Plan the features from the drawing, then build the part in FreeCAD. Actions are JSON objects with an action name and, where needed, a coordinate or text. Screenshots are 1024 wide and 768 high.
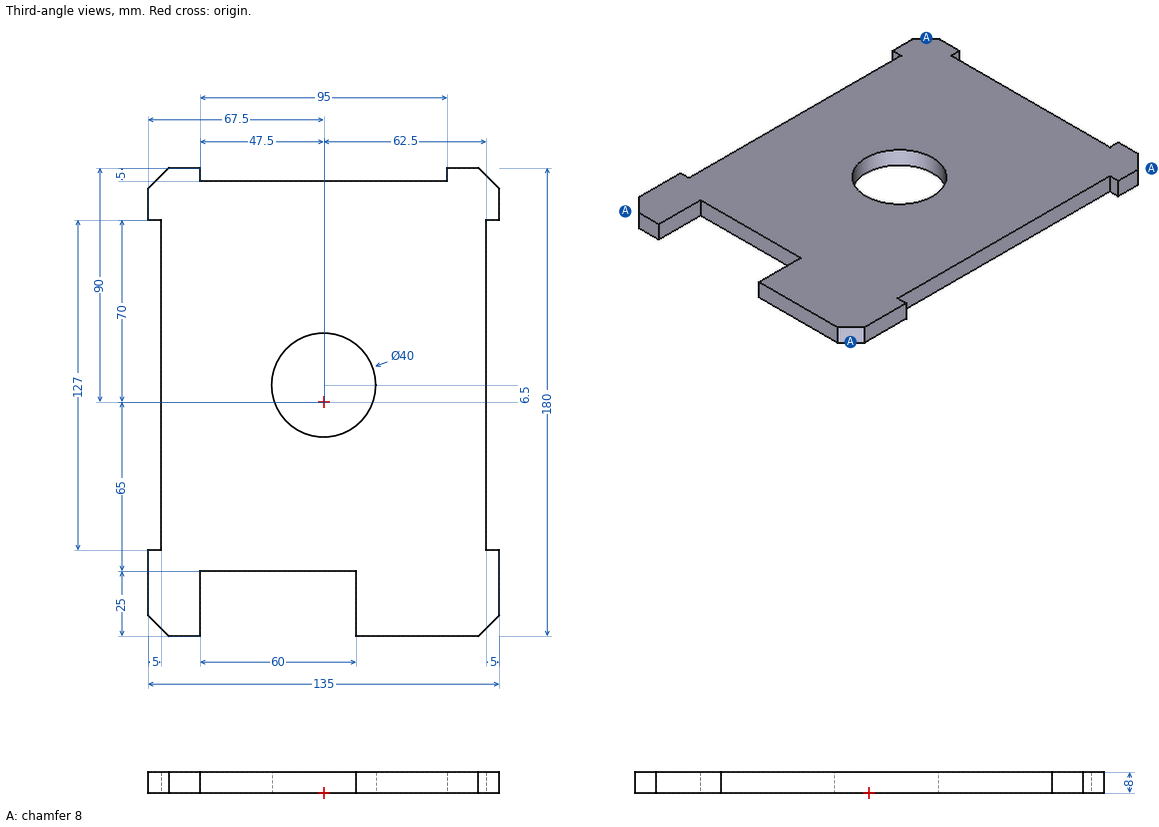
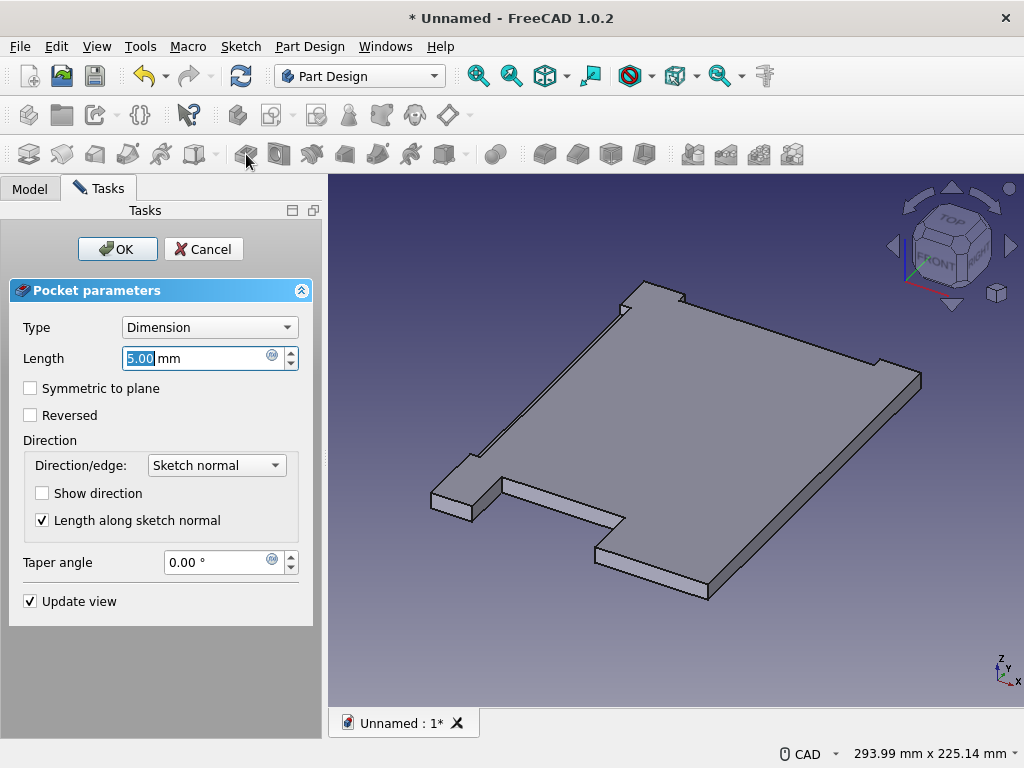
{"action": "left_click", "coordinate": [210, 328]}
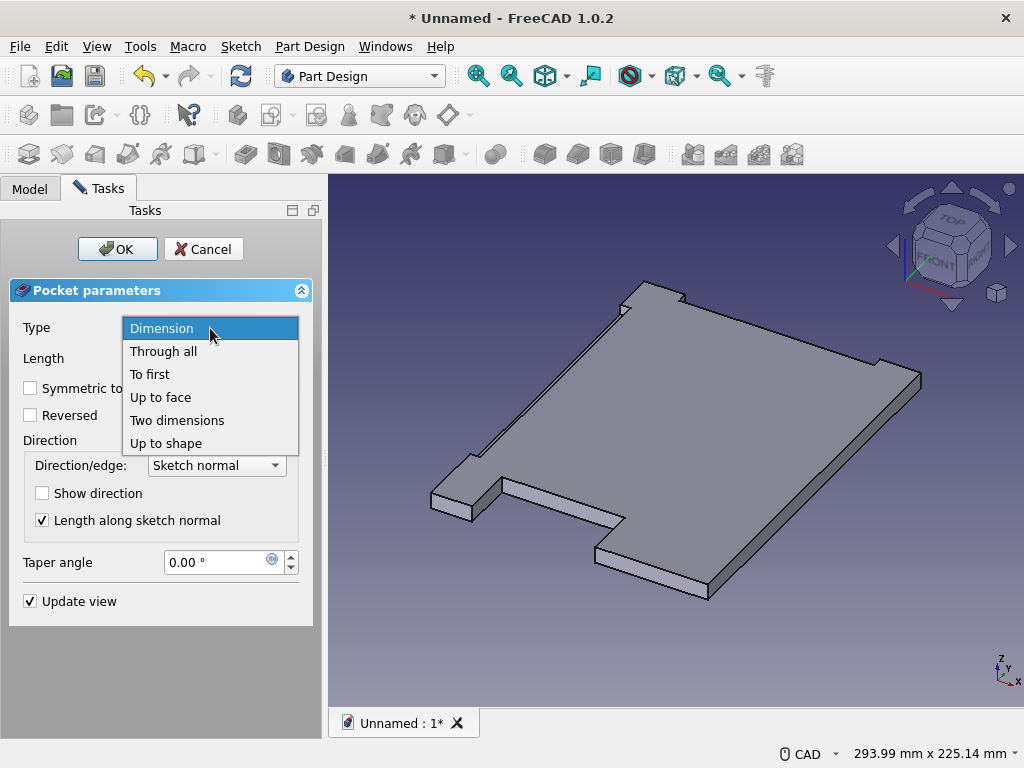
{"action": "left_click", "coordinate": [208, 374]}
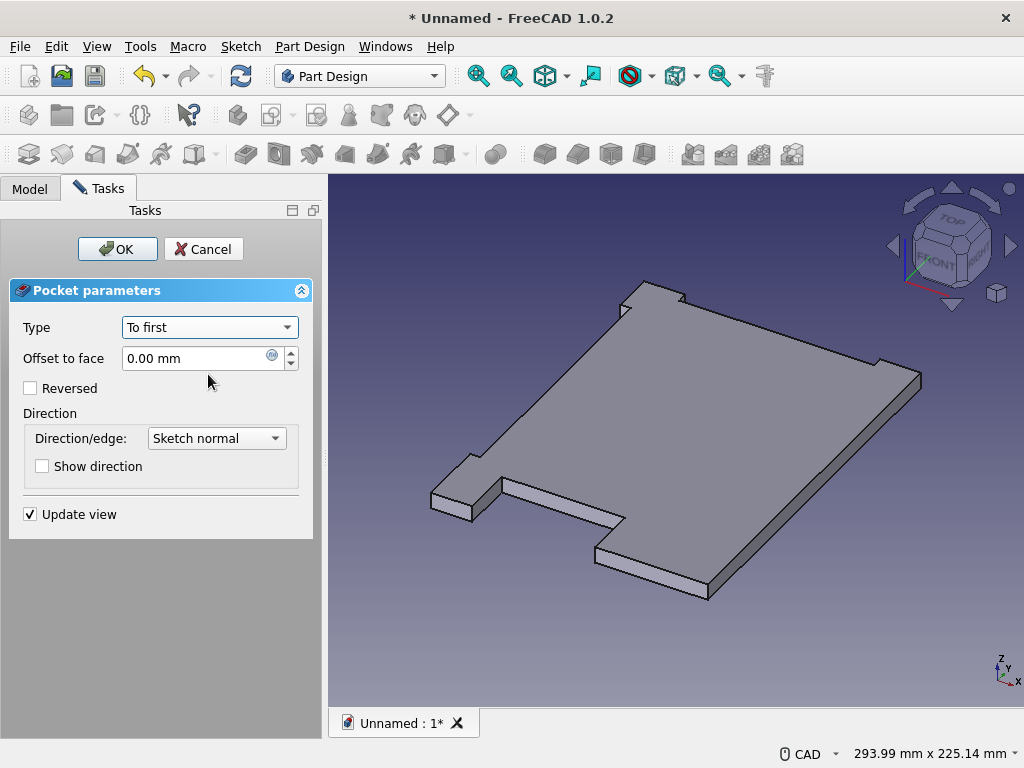
{"action": "left_click", "coordinate": [118, 249]}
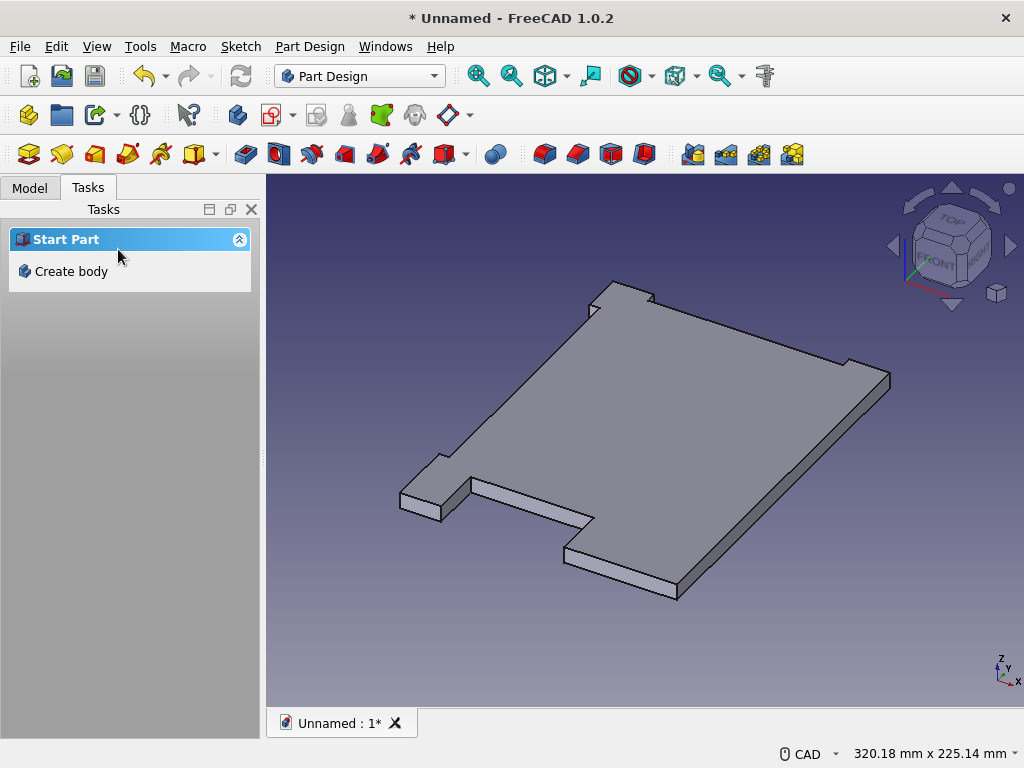
{"action": "left_click", "coordinate": [645, 432]}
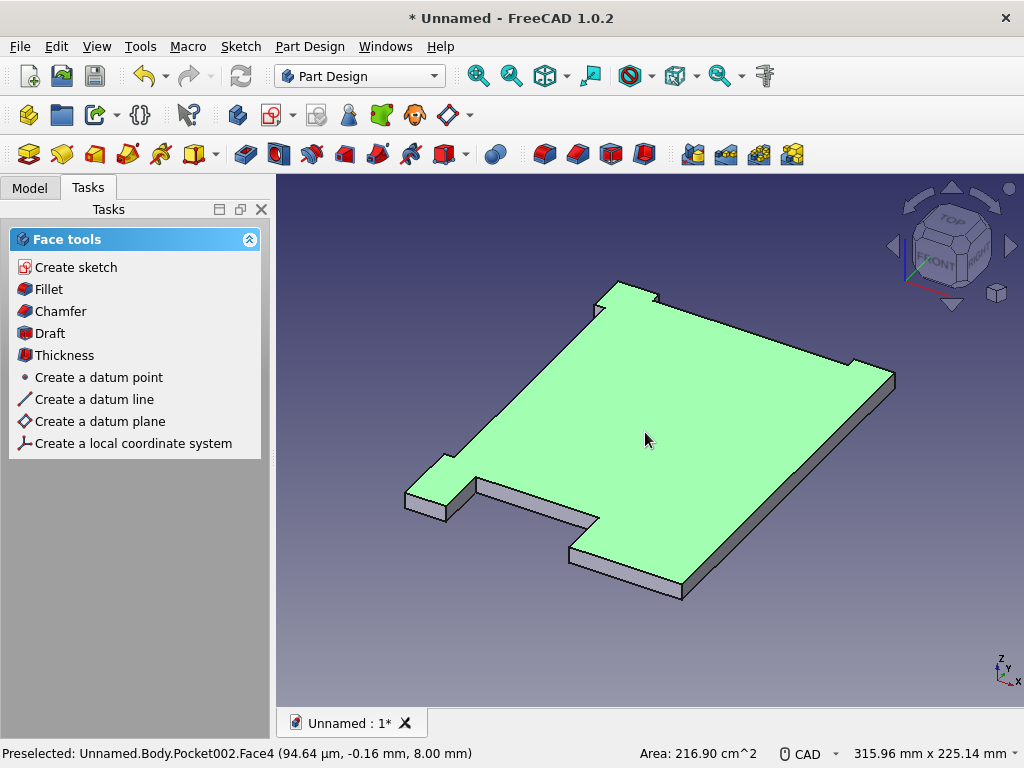
{"action": "left_click", "coordinate": [270, 116]}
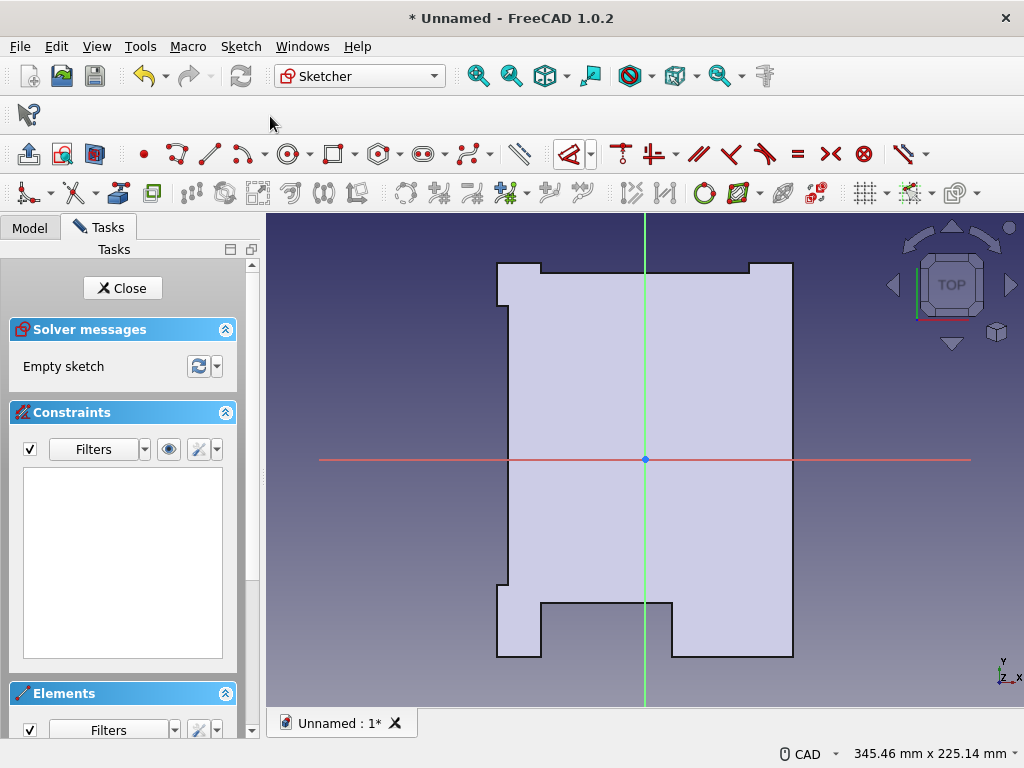
{"action": "key", "text": "g r"}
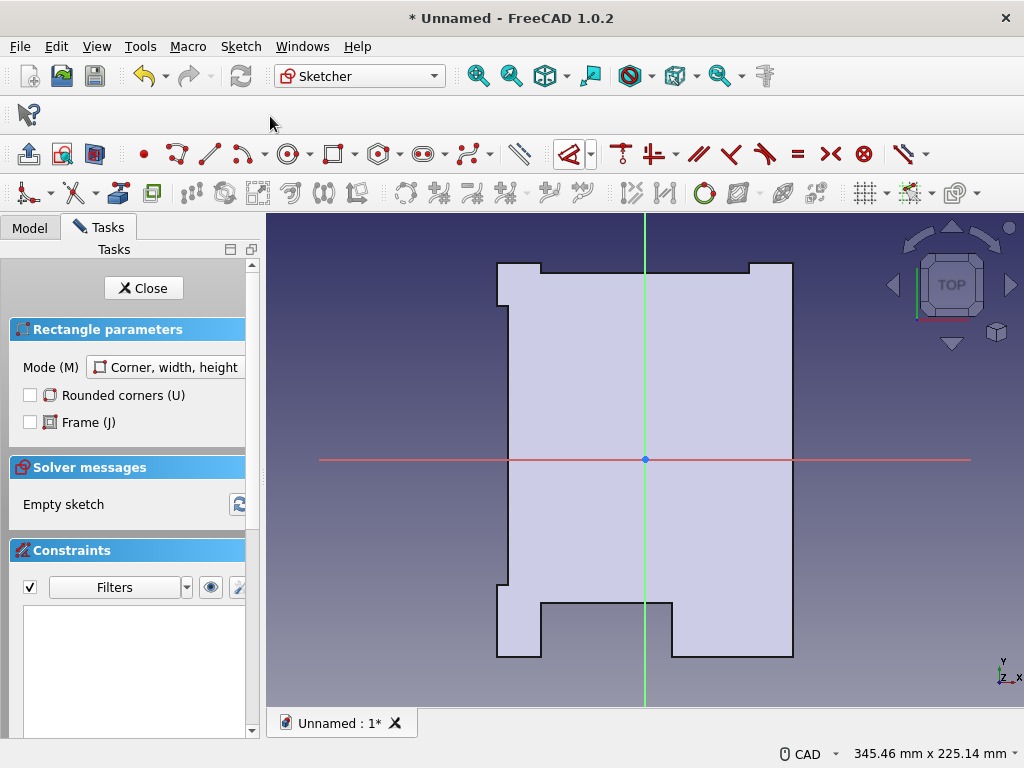
{"action": "scroll", "coordinate": [782, 306], "scroll_direction": "up", "scroll_amount": 2}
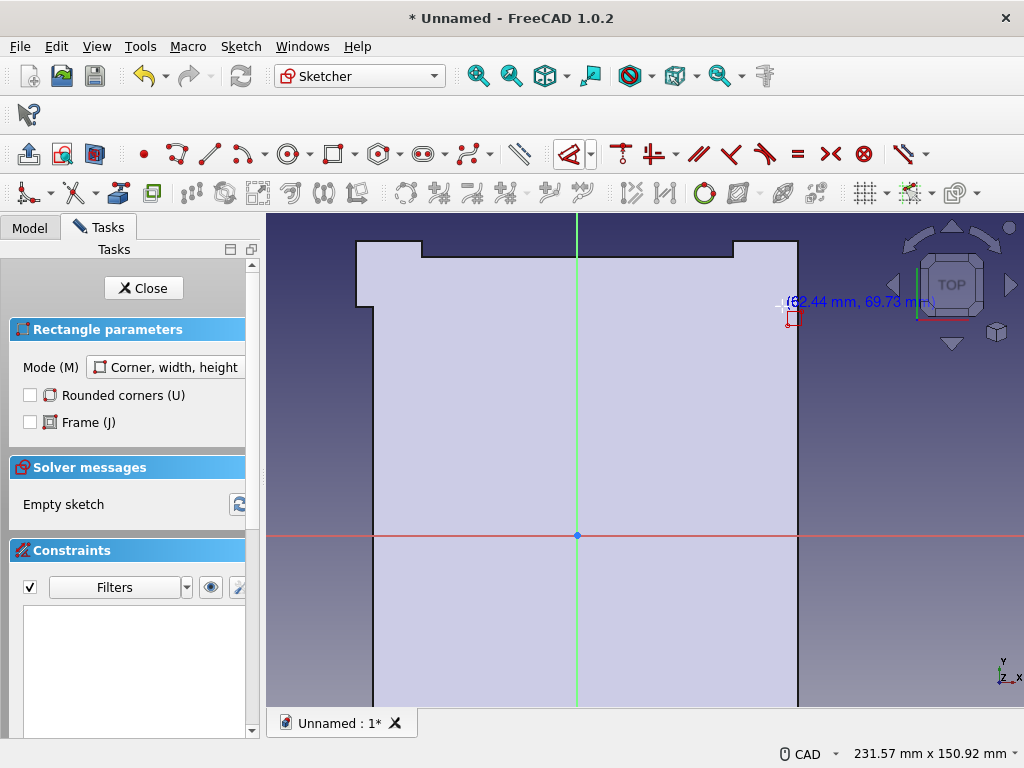
{"action": "left_click", "coordinate": [782, 307]}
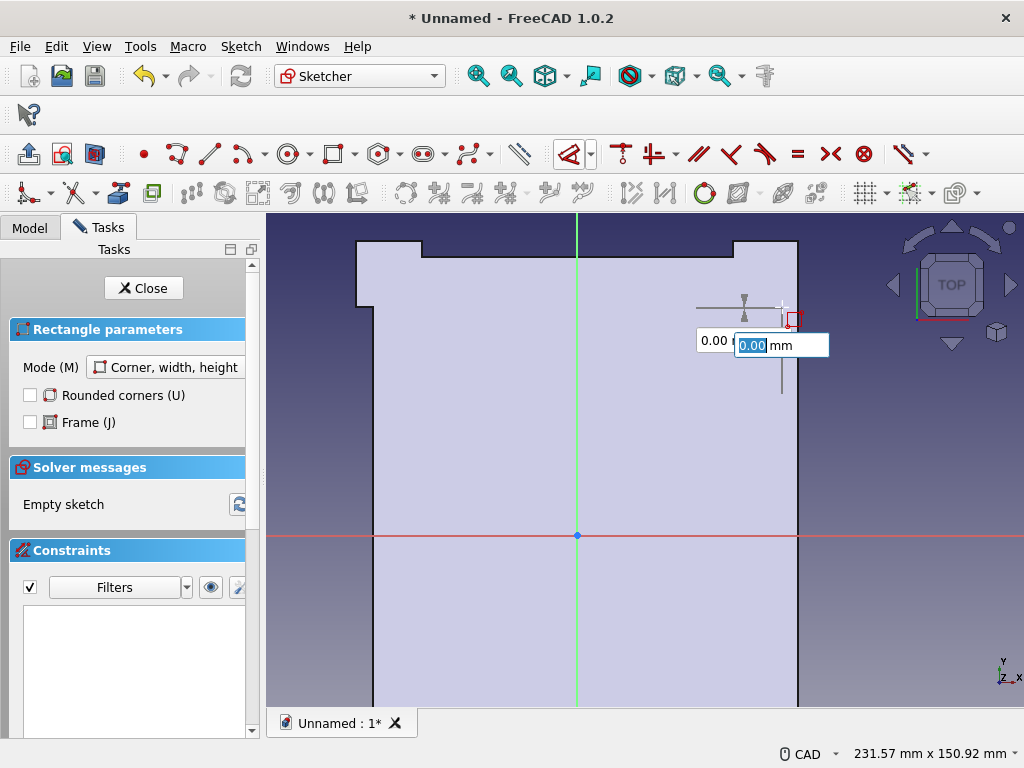
{"action": "scroll", "coordinate": [294, 241], "scroll_direction": "down", "scroll_amount": 1}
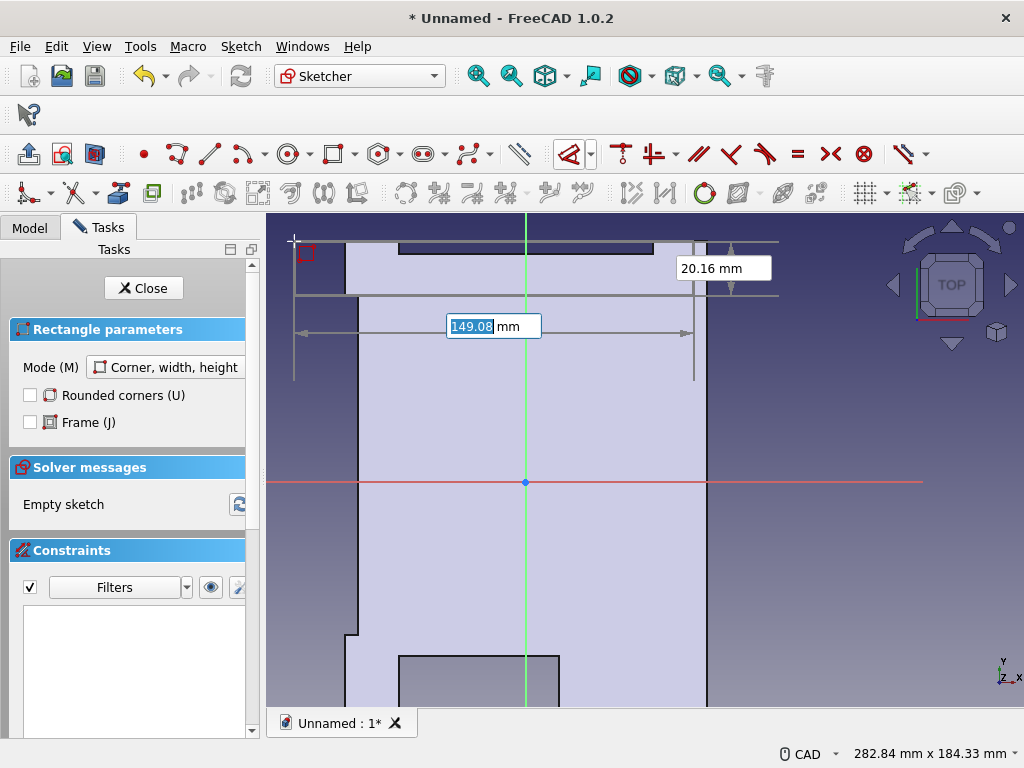
{"action": "left_click", "coordinate": [707, 635]}
{"action": "key", "text": "Escape"}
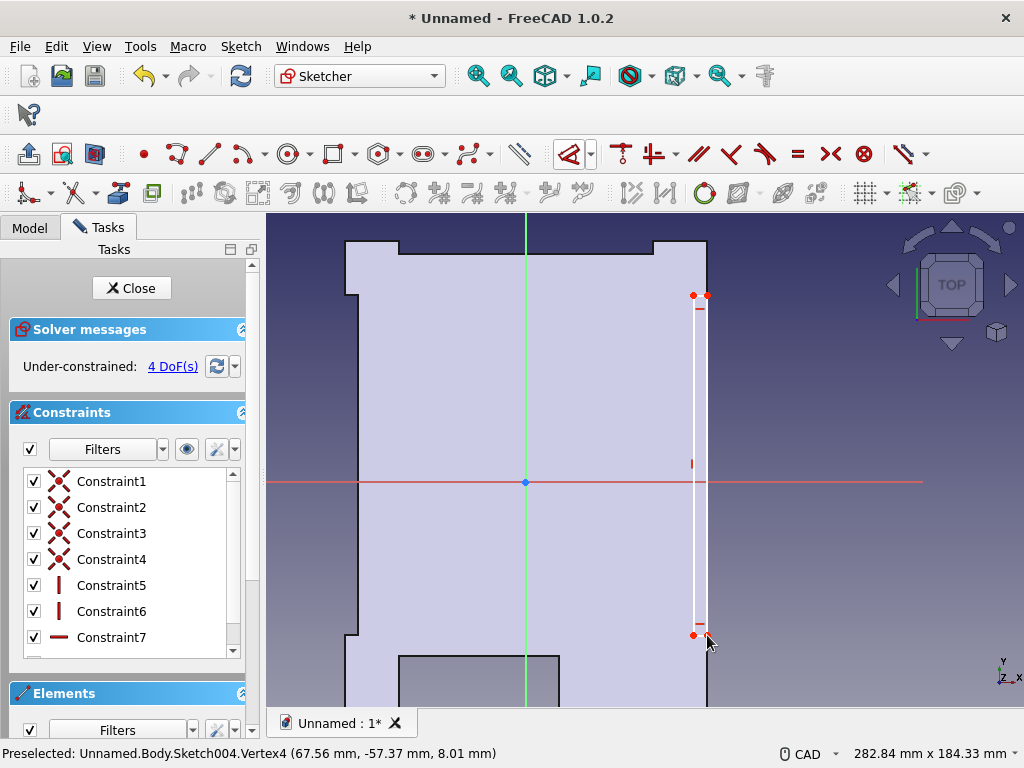
{"action": "scroll", "coordinate": [700, 636], "scroll_direction": "up", "scroll_amount": 6}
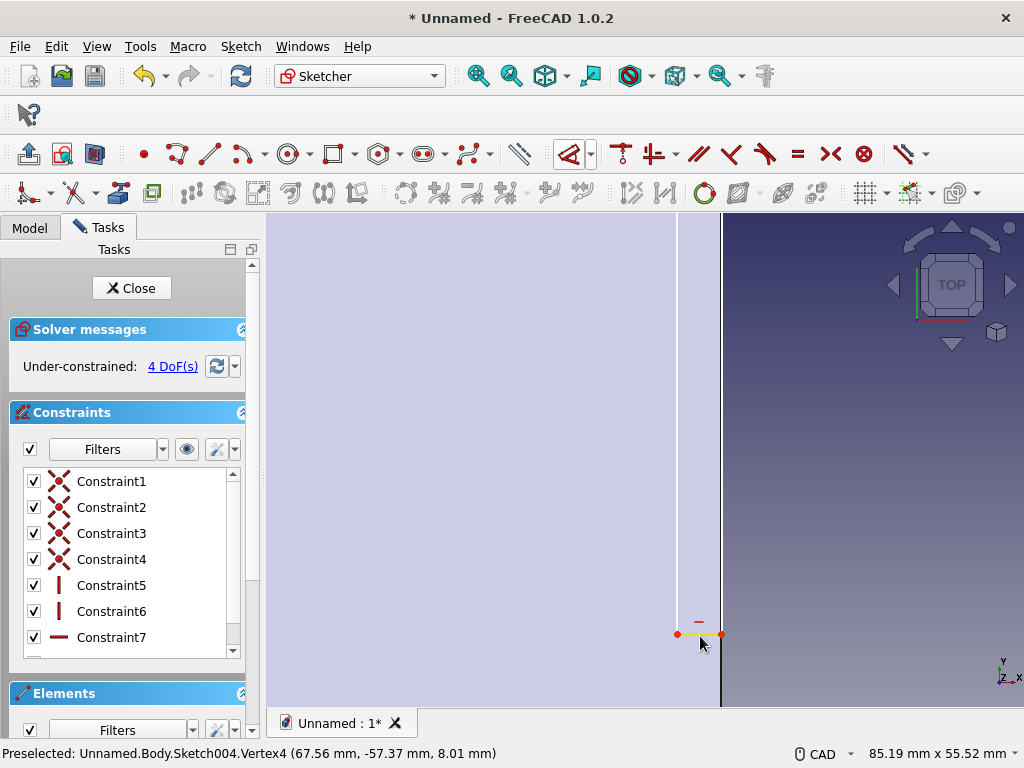
{"action": "left_click", "coordinate": [700, 634]}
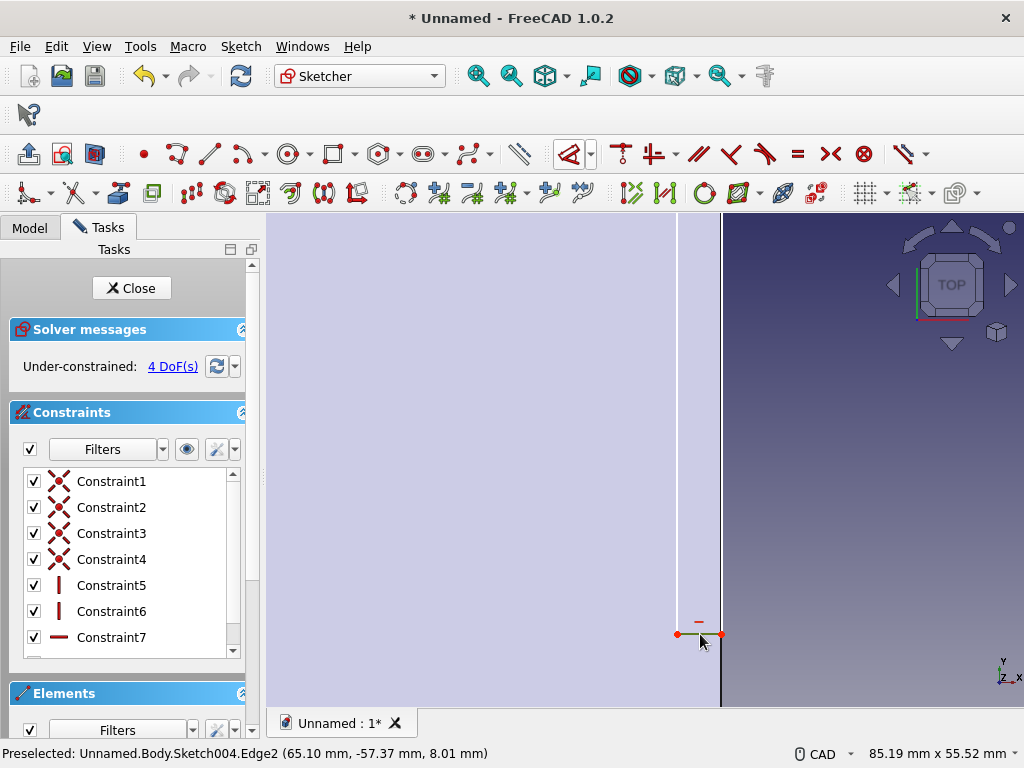
{"action": "key", "text": "l"}